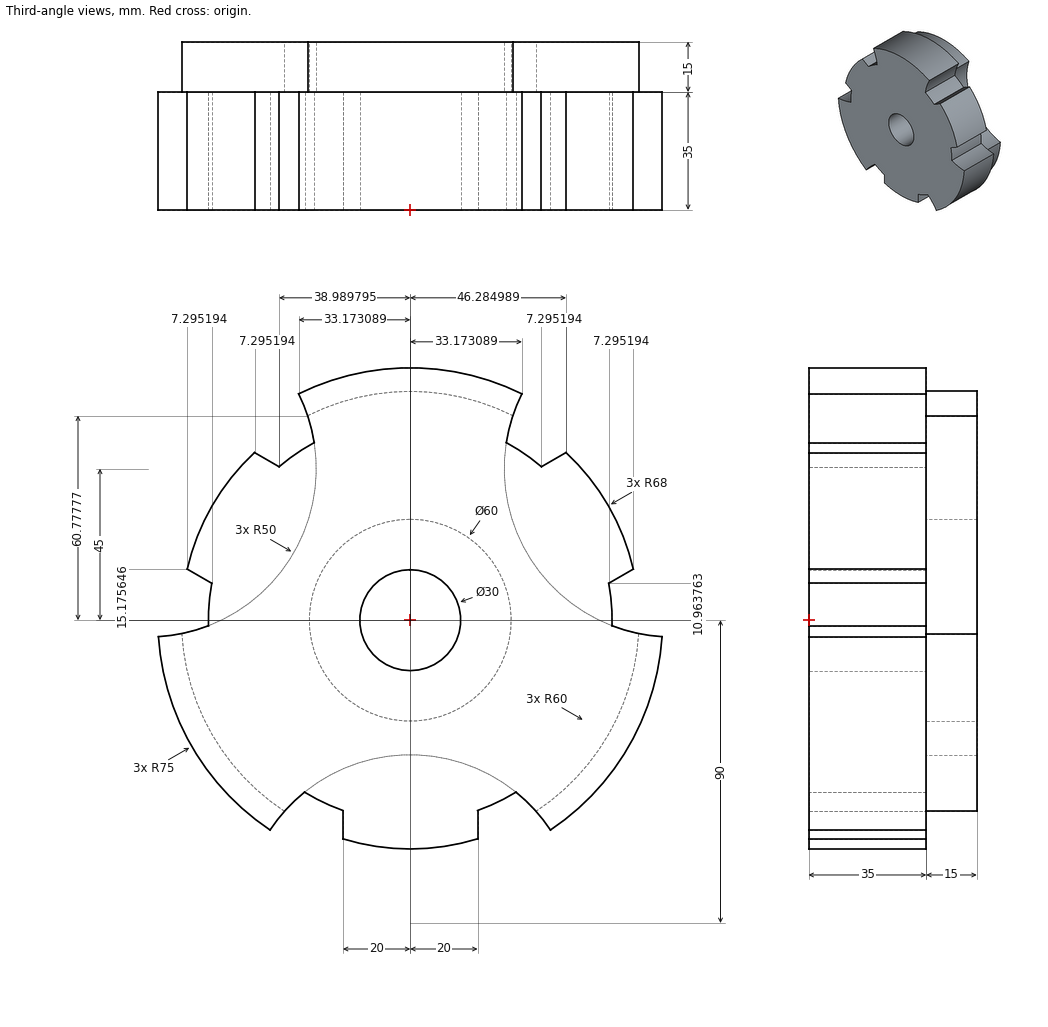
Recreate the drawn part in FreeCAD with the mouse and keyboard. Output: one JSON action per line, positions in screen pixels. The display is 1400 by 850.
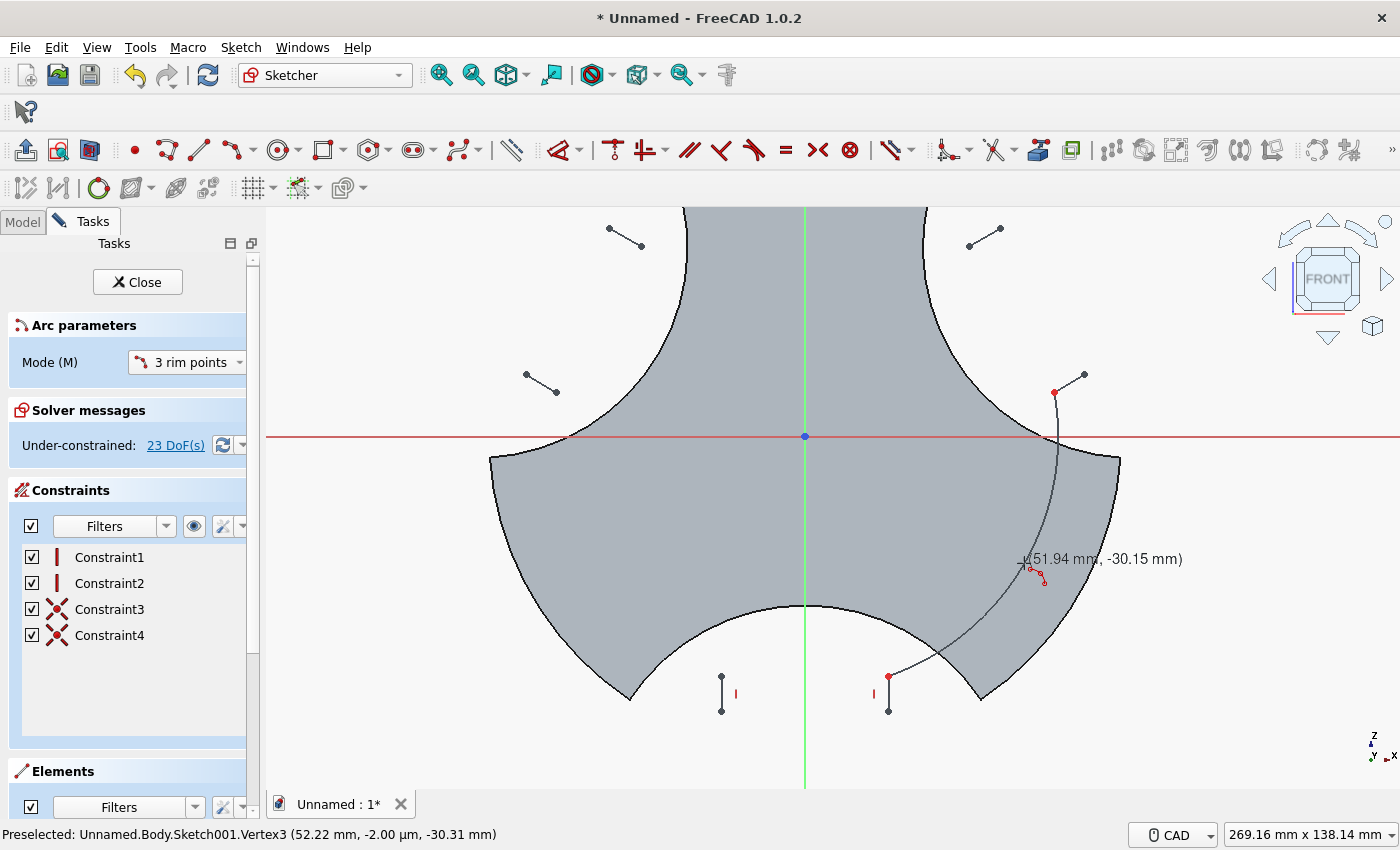
{"action": "left_click", "coordinate": [1084, 375]}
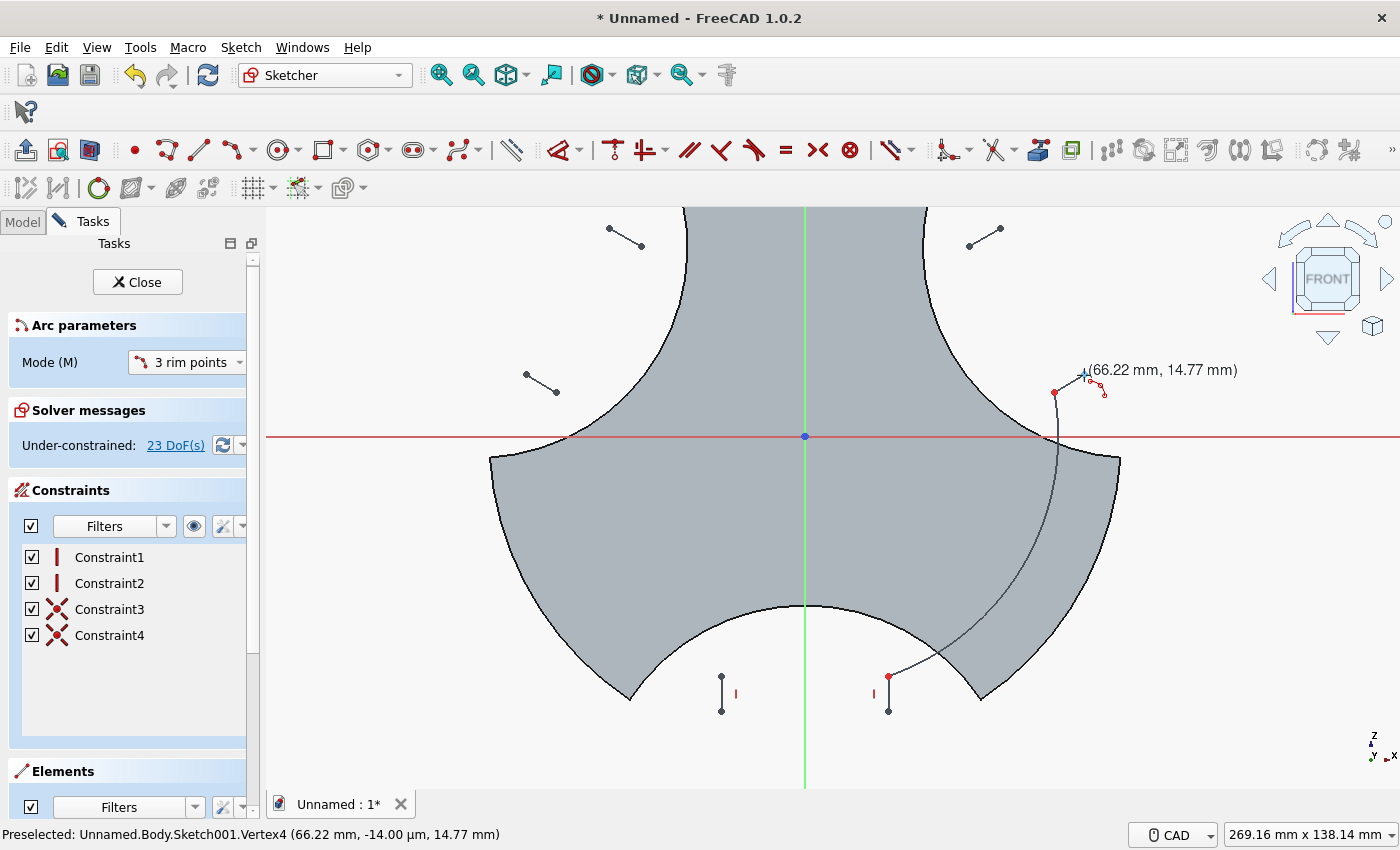
{"action": "scroll", "coordinate": [682, 588], "scroll_direction": "down", "scroll_amount": 2}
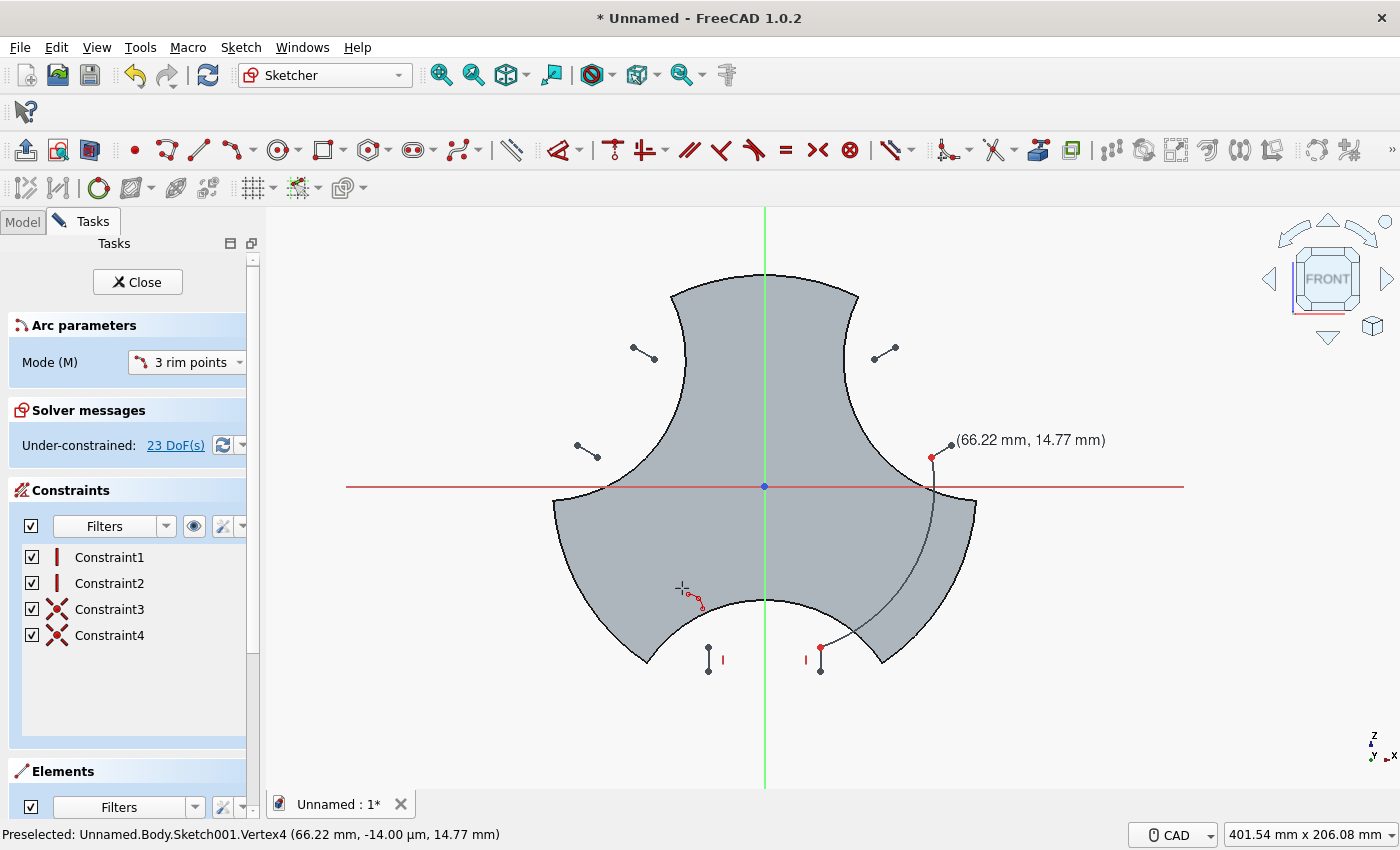
{"action": "scroll", "coordinate": [895, 346], "scroll_direction": "up", "scroll_amount": 2}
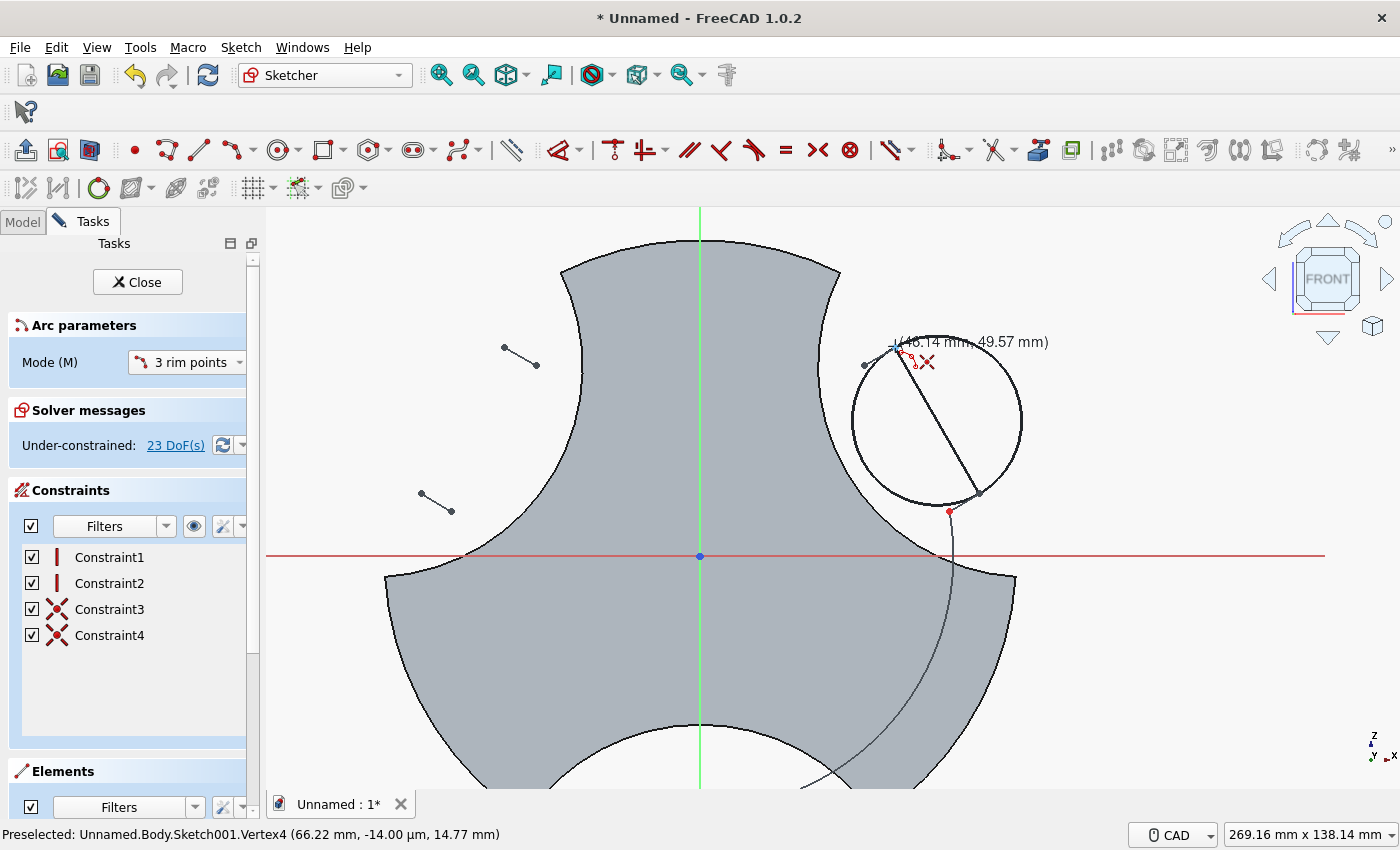
{"action": "left_click", "coordinate": [896, 348]}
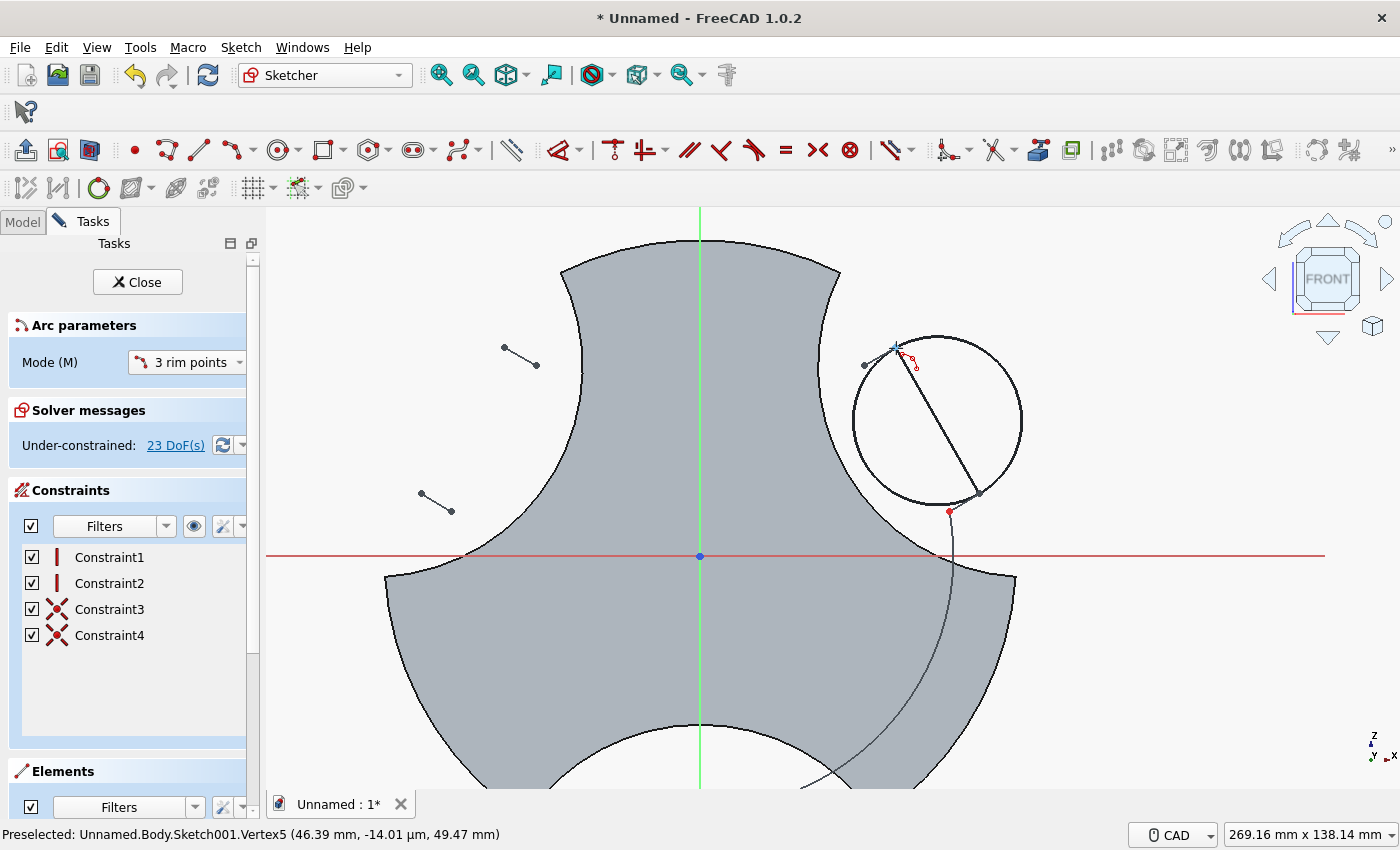
{"action": "scroll", "coordinate": [948, 413], "scroll_direction": "up", "scroll_amount": 2}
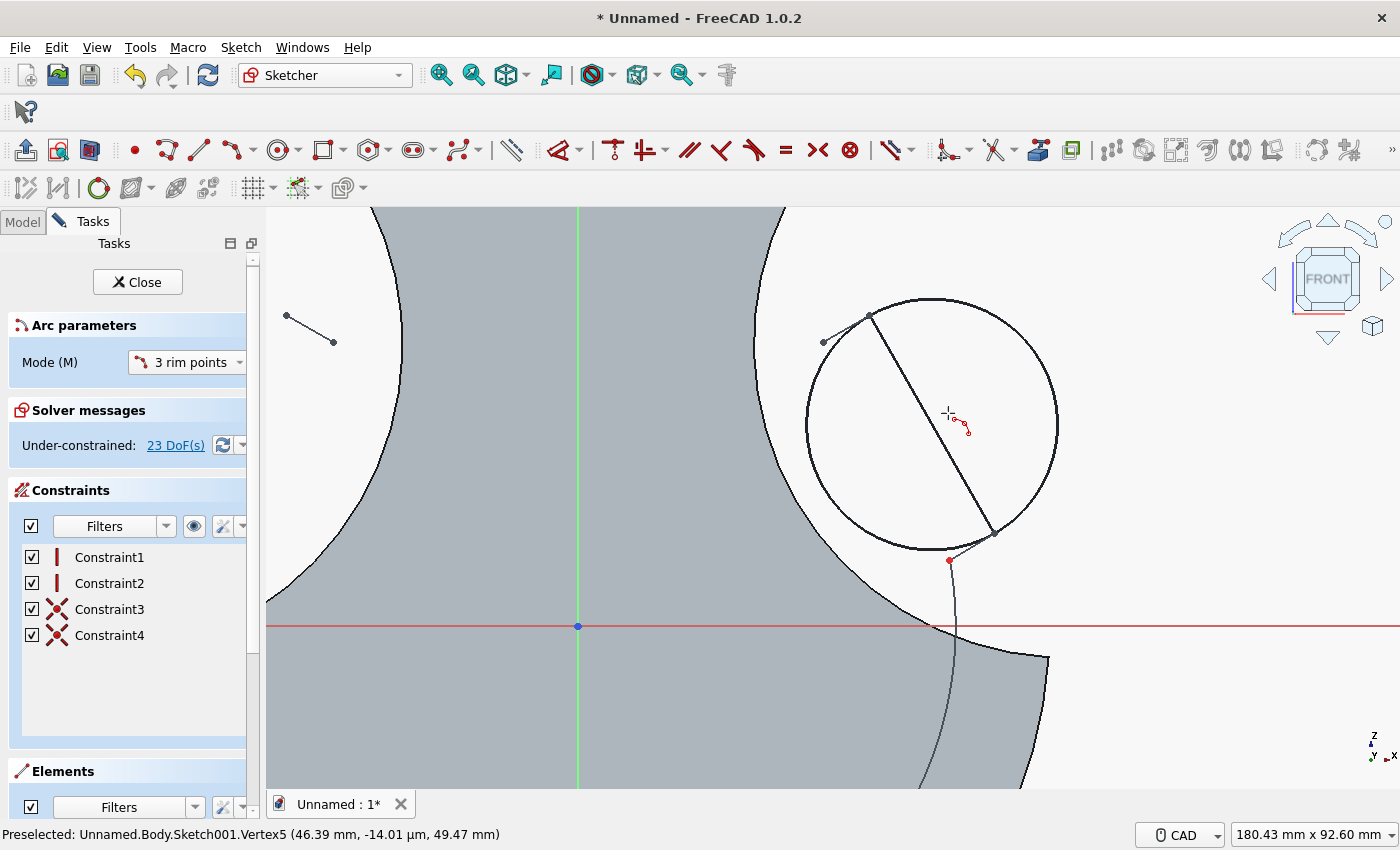
{"action": "left_click", "coordinate": [948, 413]}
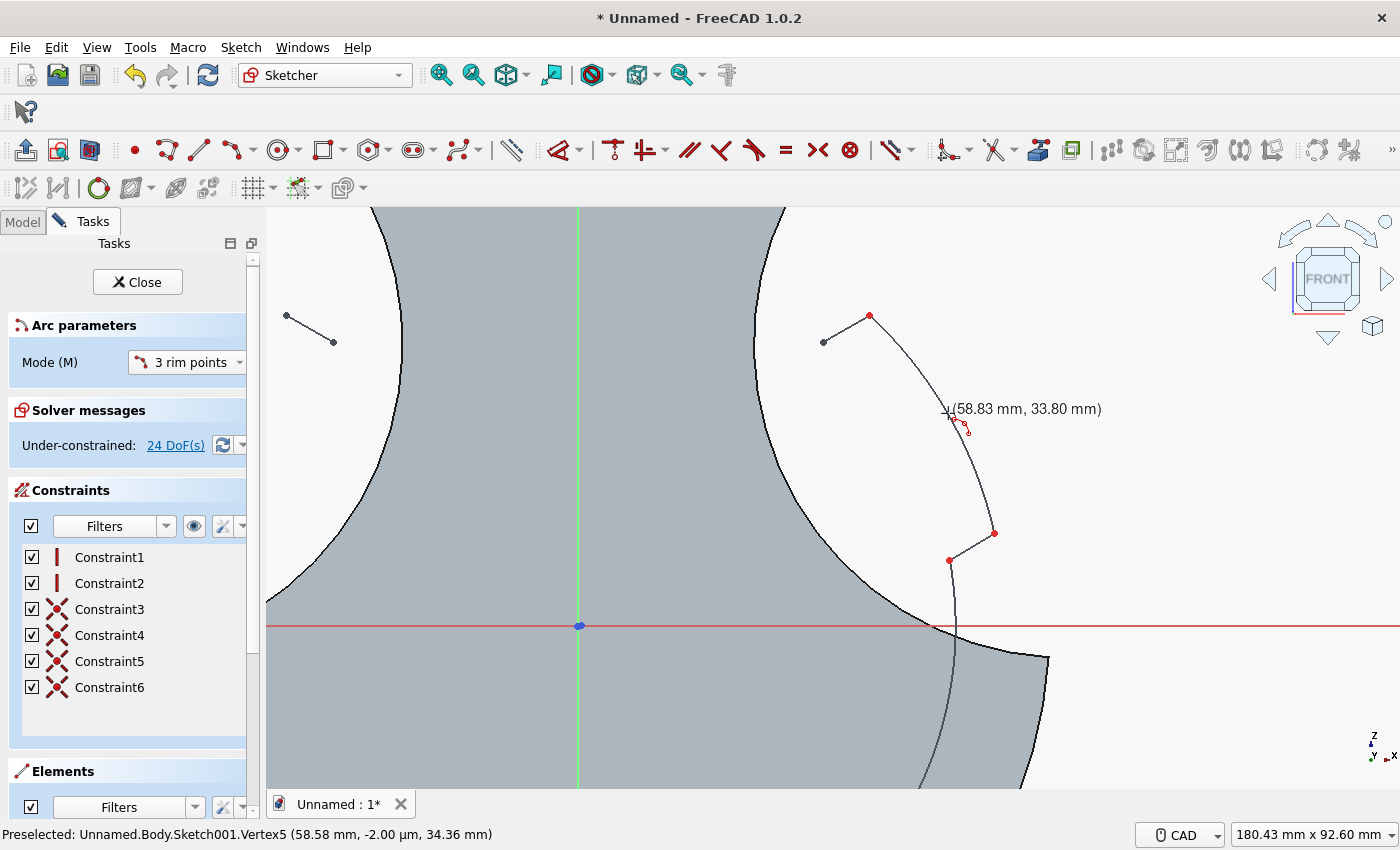
{"action": "left_click", "coordinate": [823, 342]}
{"action": "left_click", "coordinate": [333, 342]}
{"action": "left_click", "coordinate": [631, 253]}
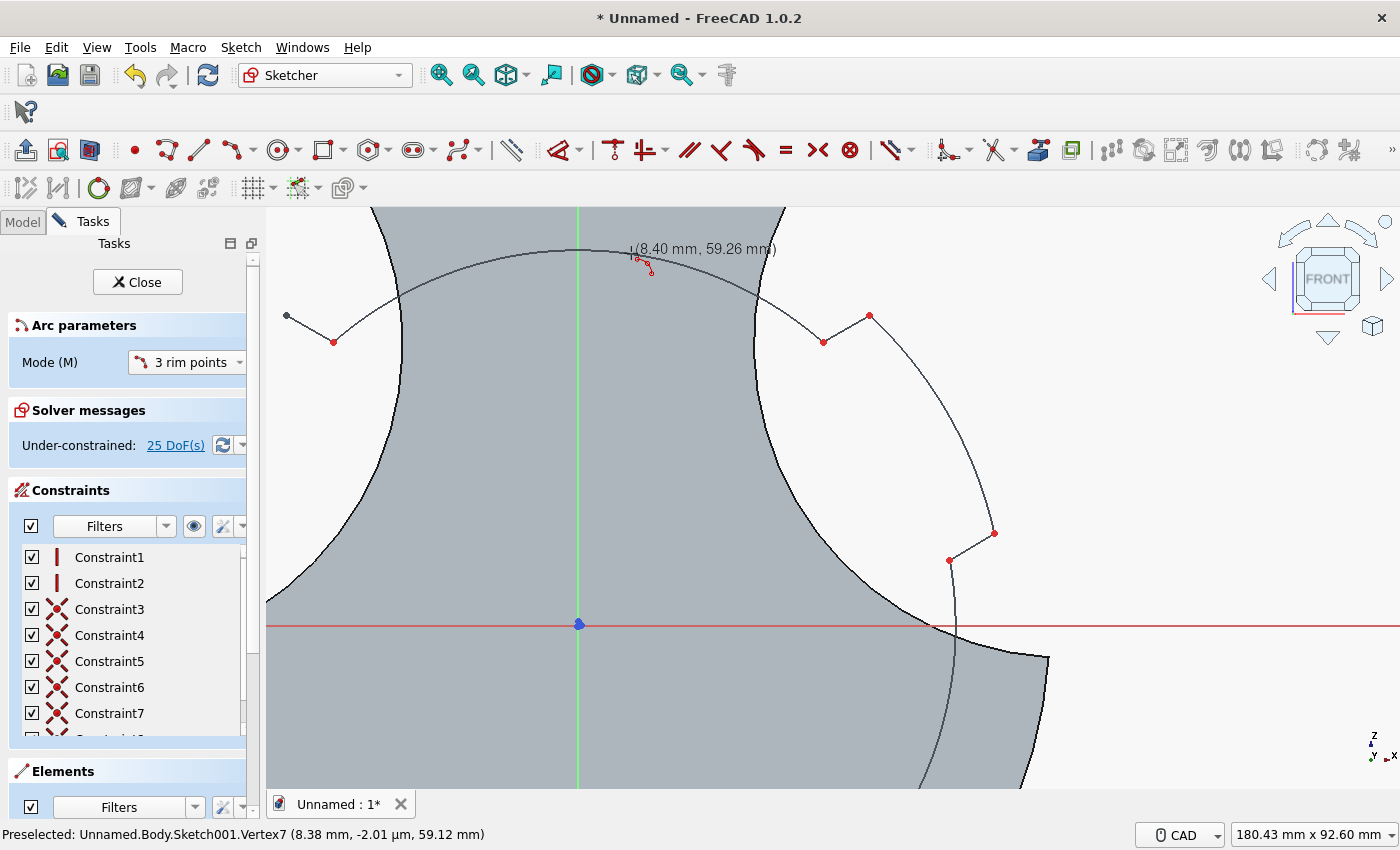
{"action": "scroll", "coordinate": [916, 373], "scroll_direction": "down", "scroll_amount": 4}